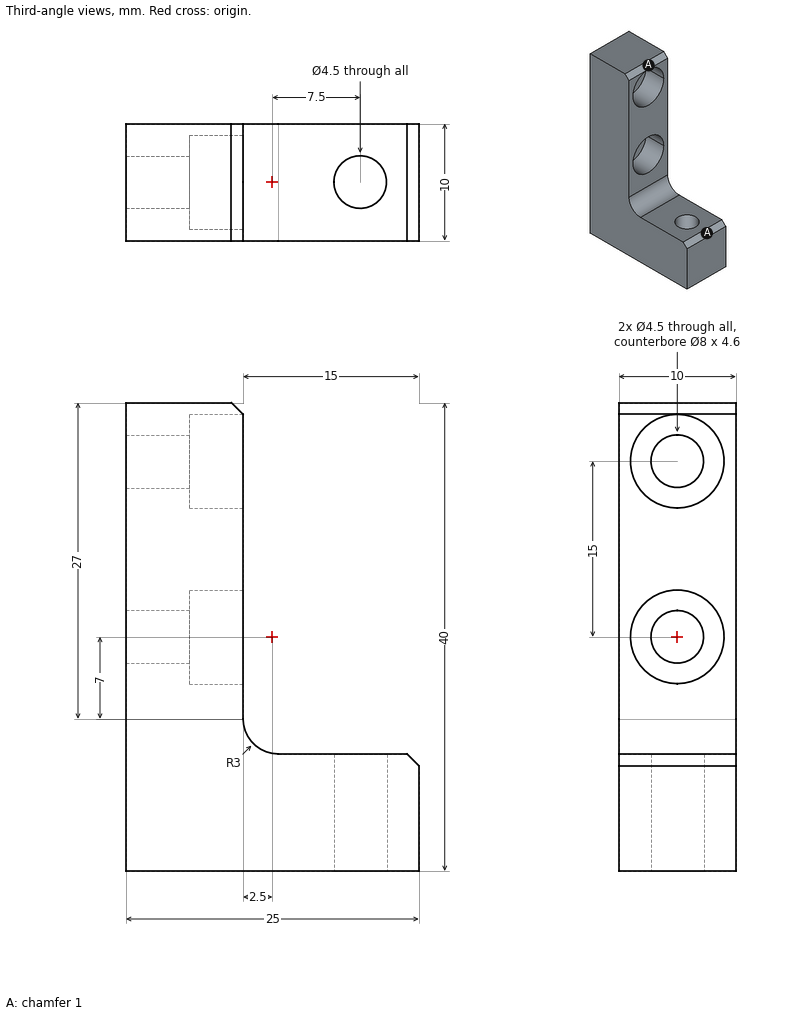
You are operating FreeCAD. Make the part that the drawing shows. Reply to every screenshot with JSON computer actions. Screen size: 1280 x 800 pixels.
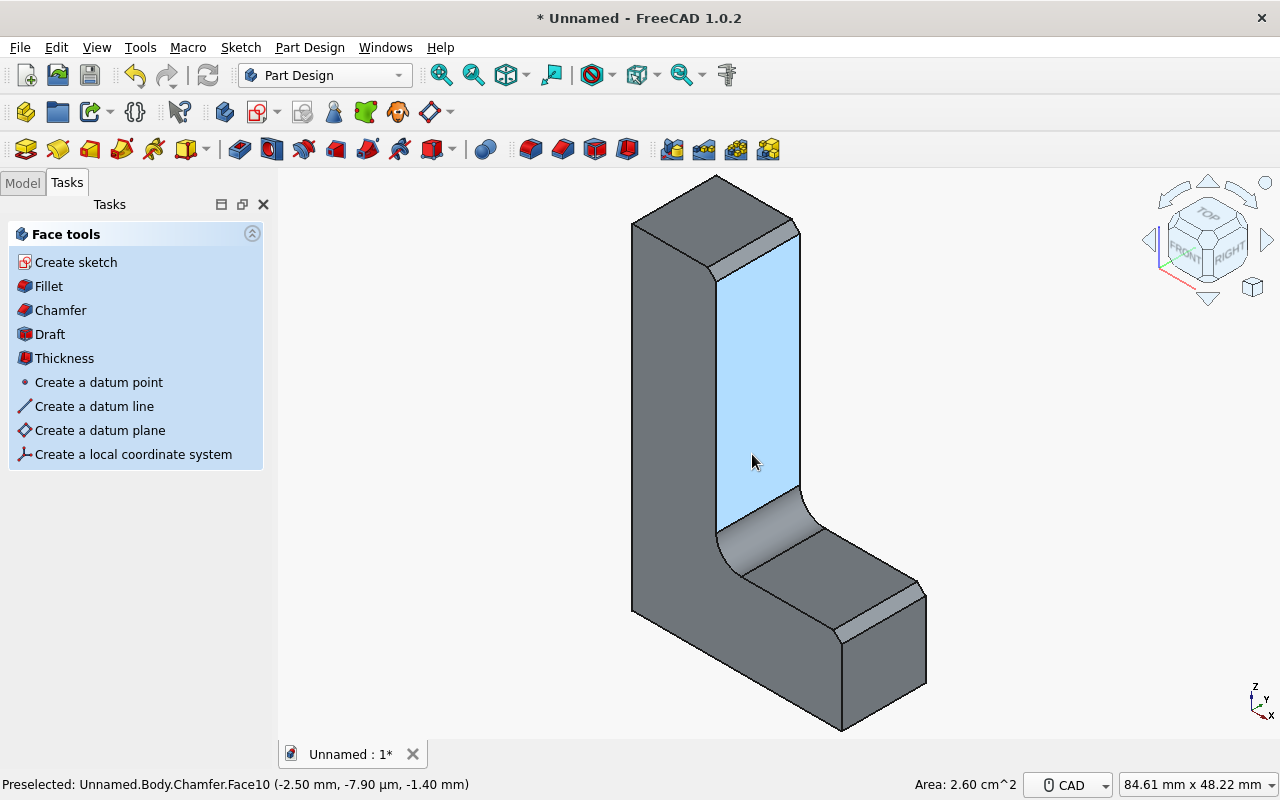
{"action": "left_click", "coordinate": [258, 112]}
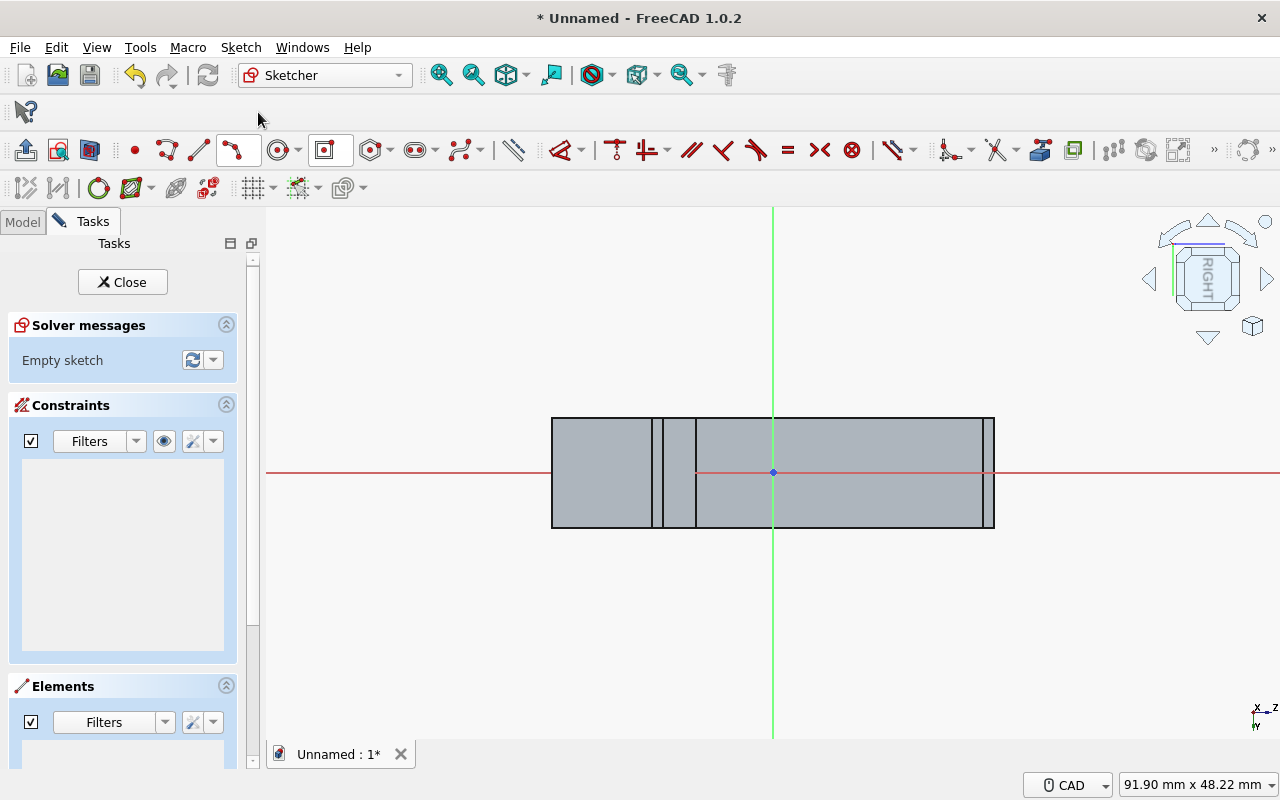
{"action": "scroll", "coordinate": [944, 473], "scroll_direction": "up", "scroll_amount": 5}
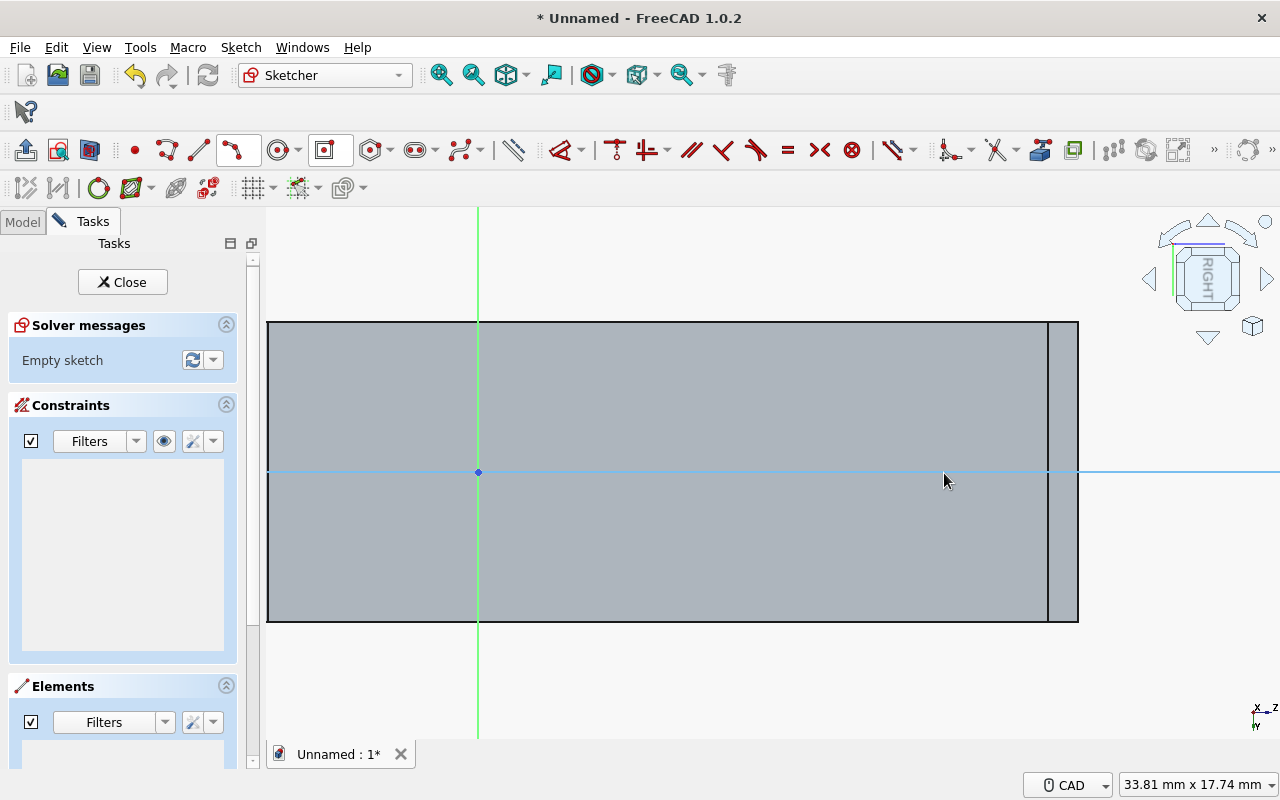
{"action": "left_click", "coordinate": [278, 150]}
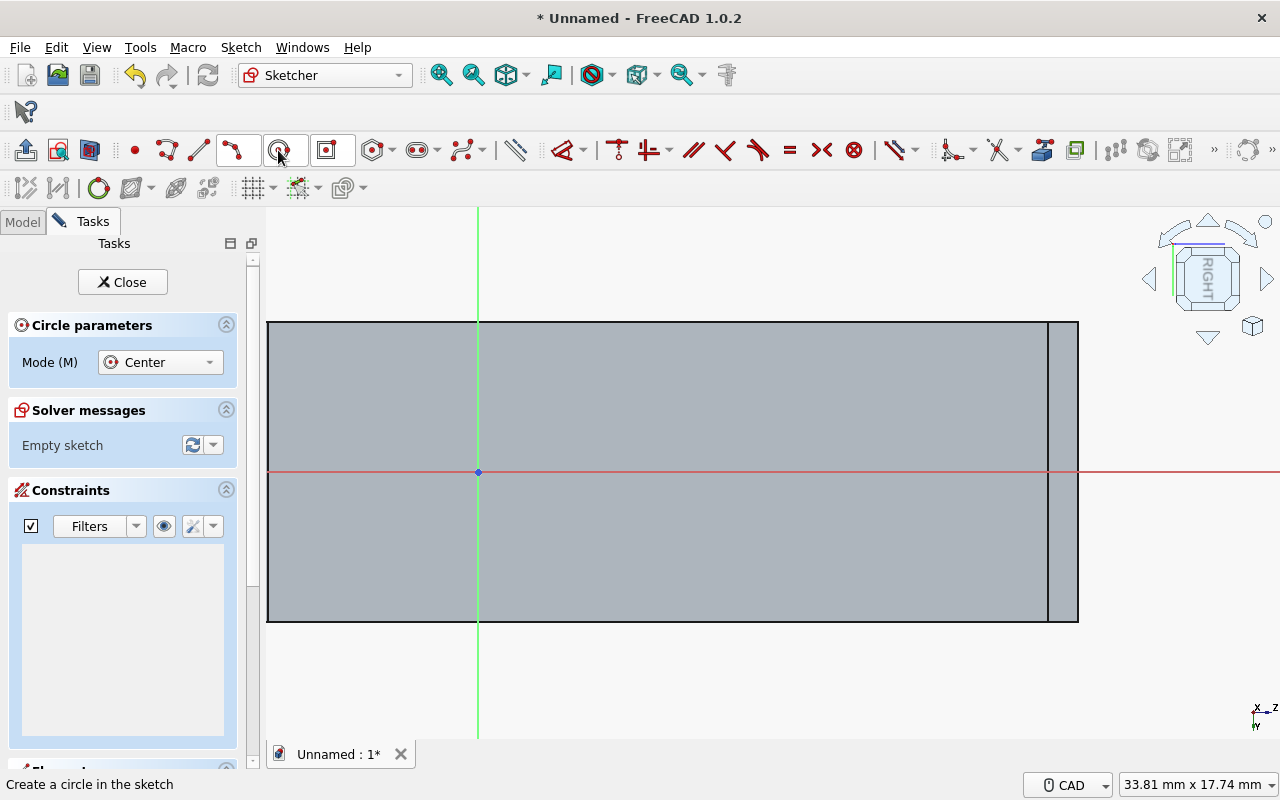
{"action": "left_click", "coordinate": [928, 472]}
{"action": "mouse_move", "coordinate": [976, 424]}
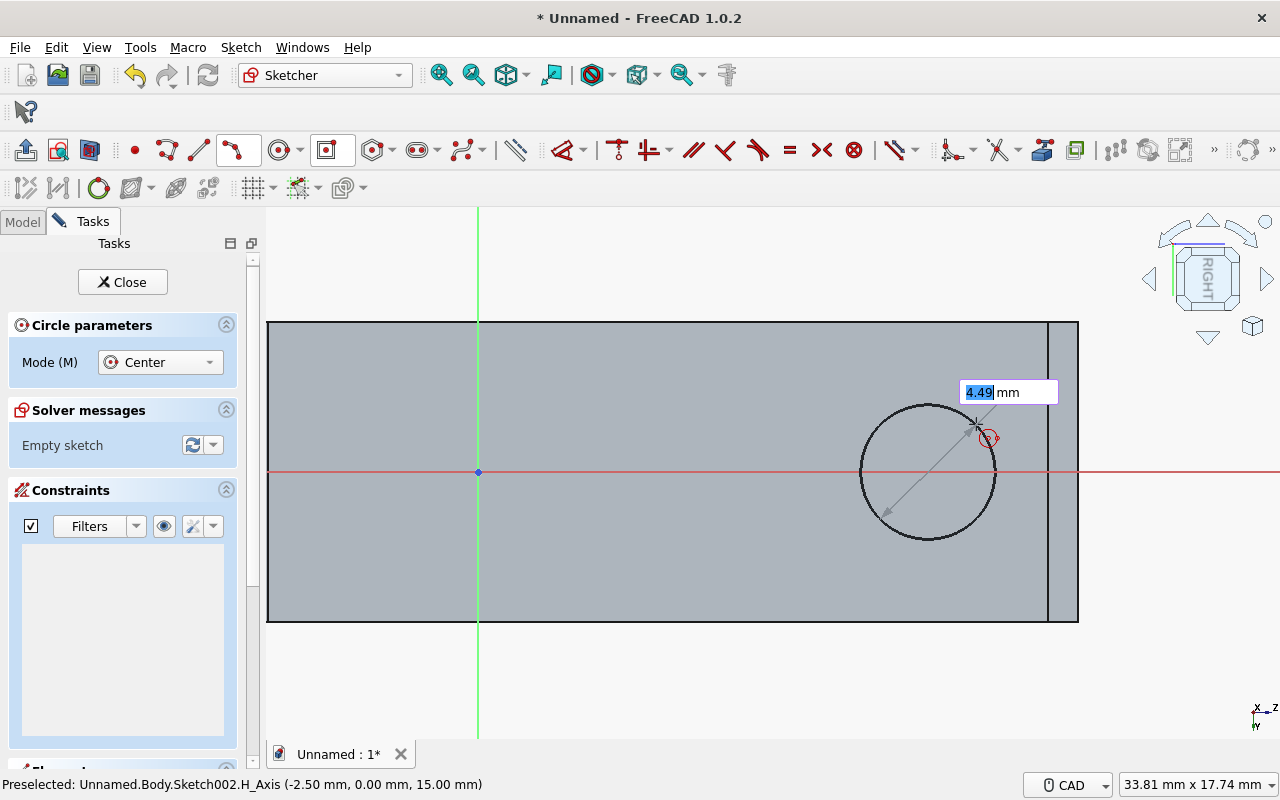
{"action": "type", "text": "4.5"}
{"action": "key", "text": "Return"}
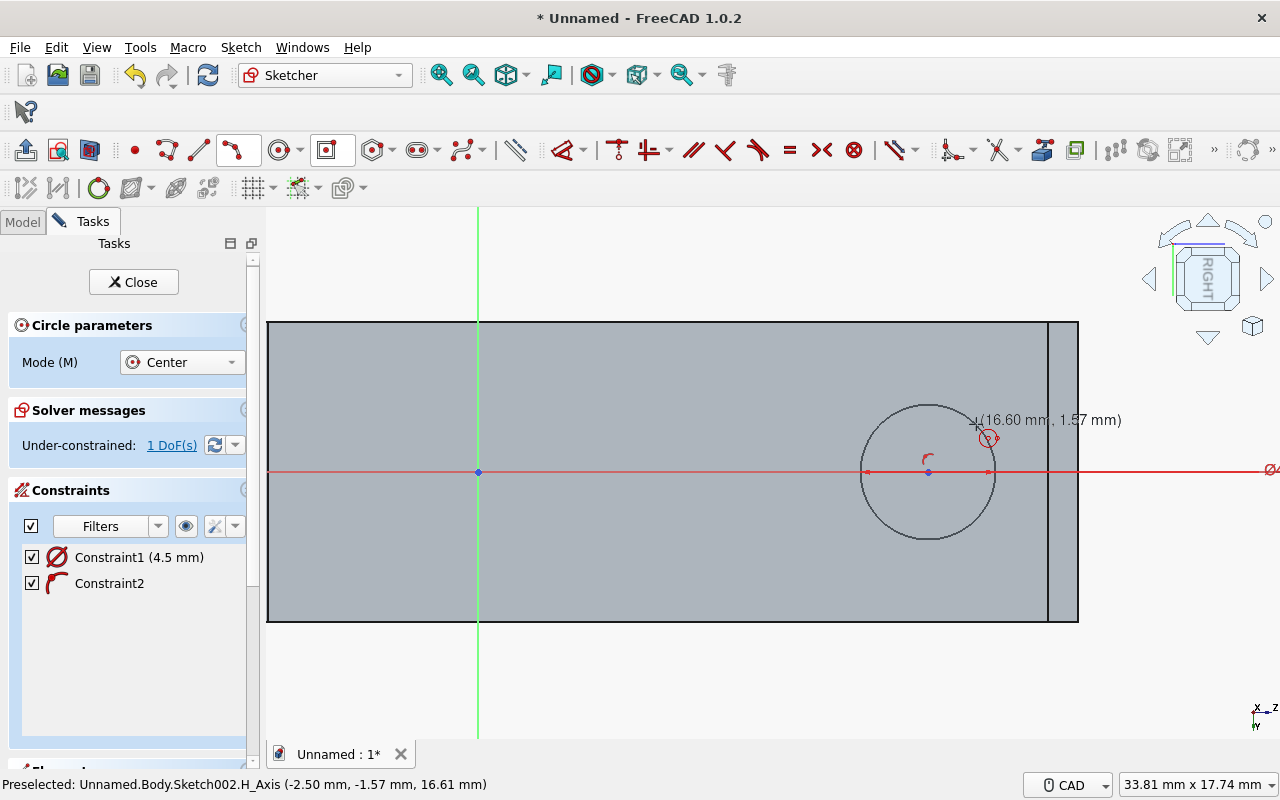
{"action": "left_click", "coordinate": [478, 472]}
{"action": "mouse_move", "coordinate": [526, 424]}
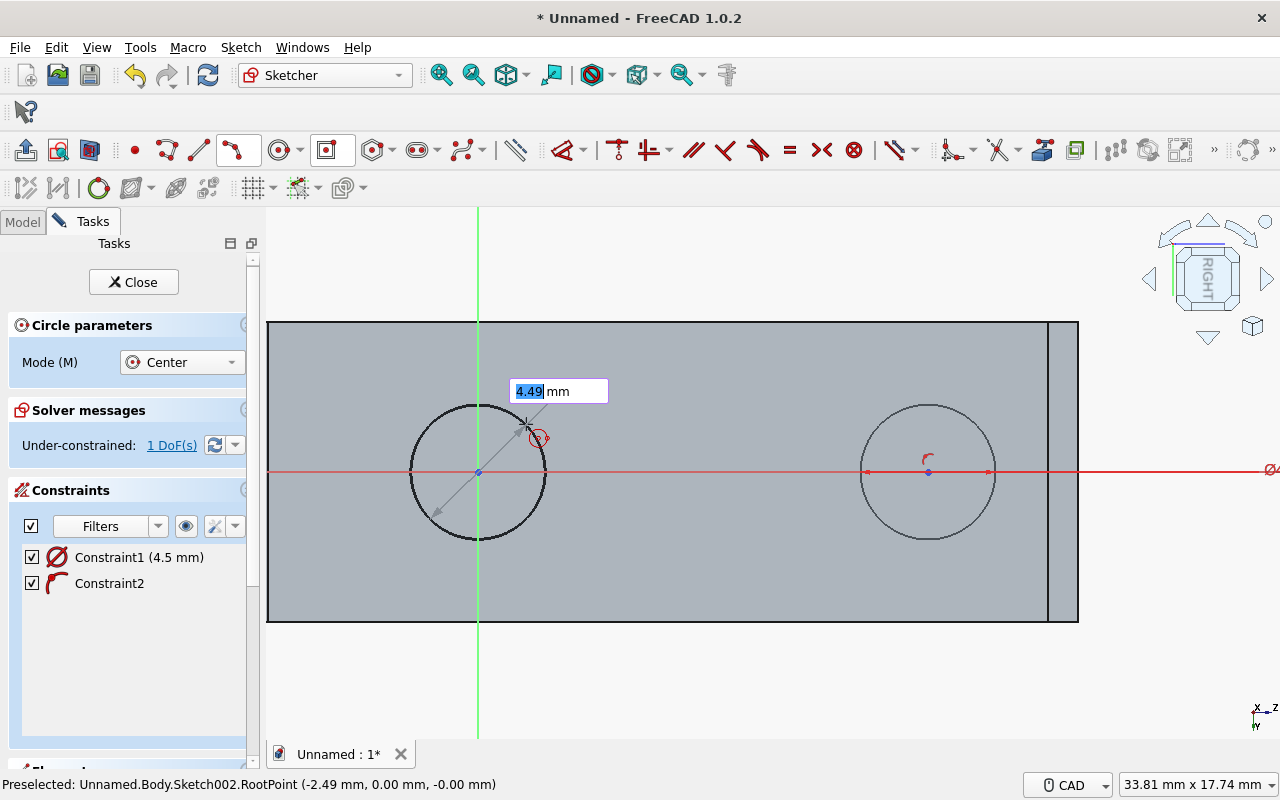
{"action": "type", "text": "4.5"}
{"action": "key", "text": "Return"}
{"action": "key", "text": "Escape"}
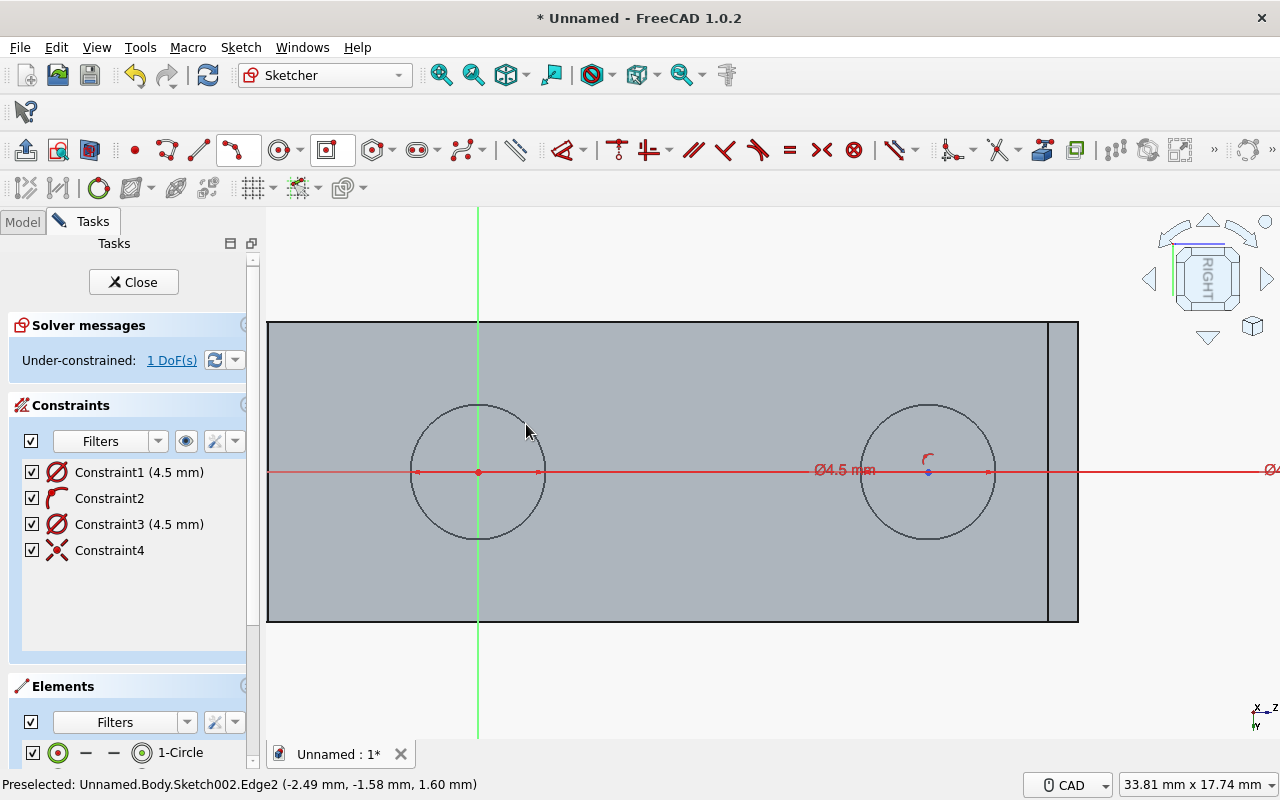
{"action": "left_click", "coordinate": [562, 150]}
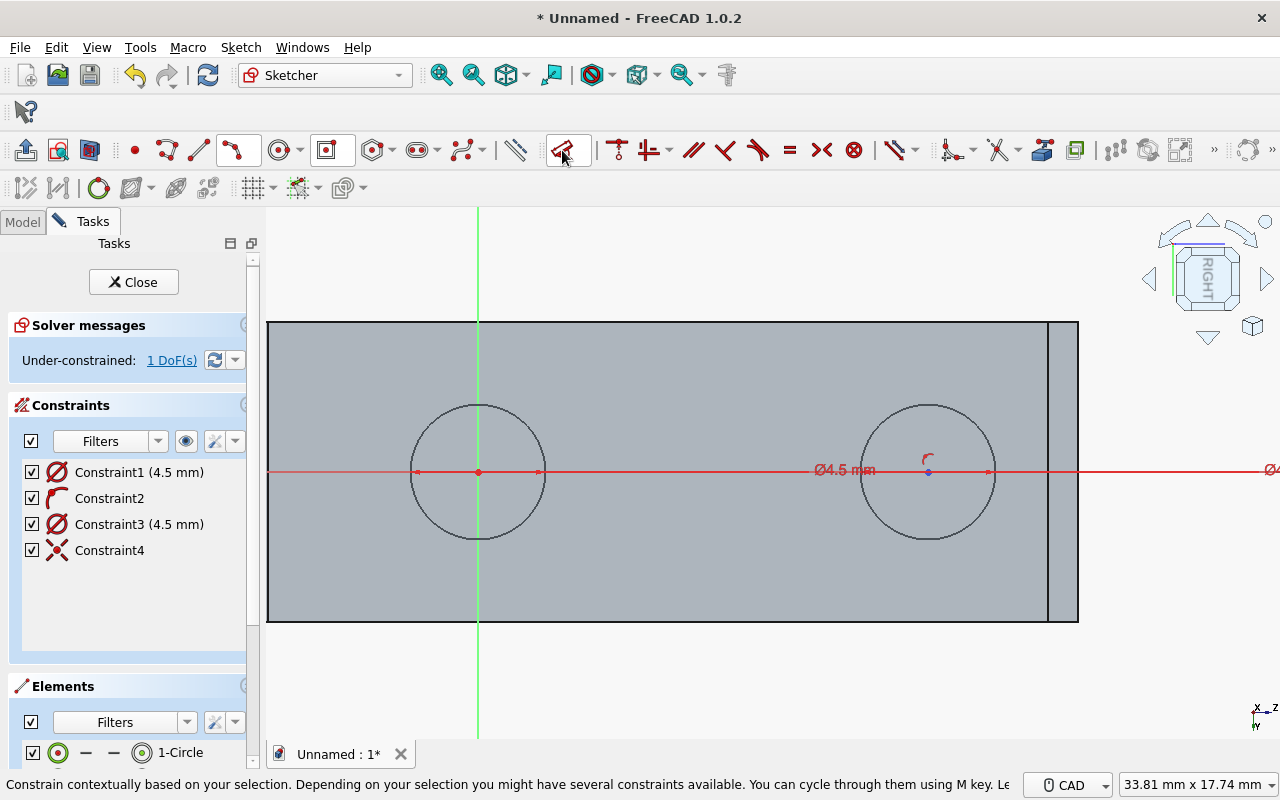
{"action": "left_click", "coordinate": [928, 472]}
{"action": "left_click", "coordinate": [703, 506]}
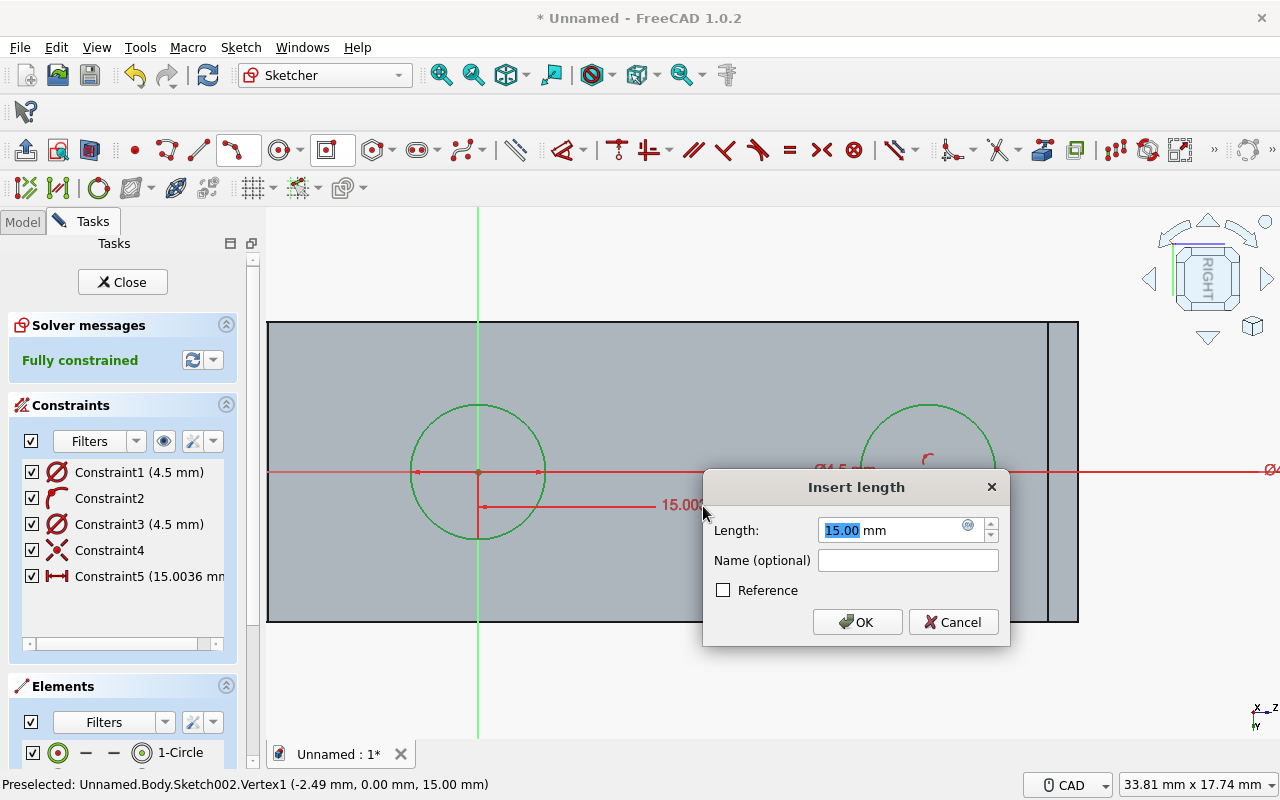
{"action": "type", "text": "15"}
{"action": "key", "text": "Return"}
{"action": "key", "text": "Escape"}